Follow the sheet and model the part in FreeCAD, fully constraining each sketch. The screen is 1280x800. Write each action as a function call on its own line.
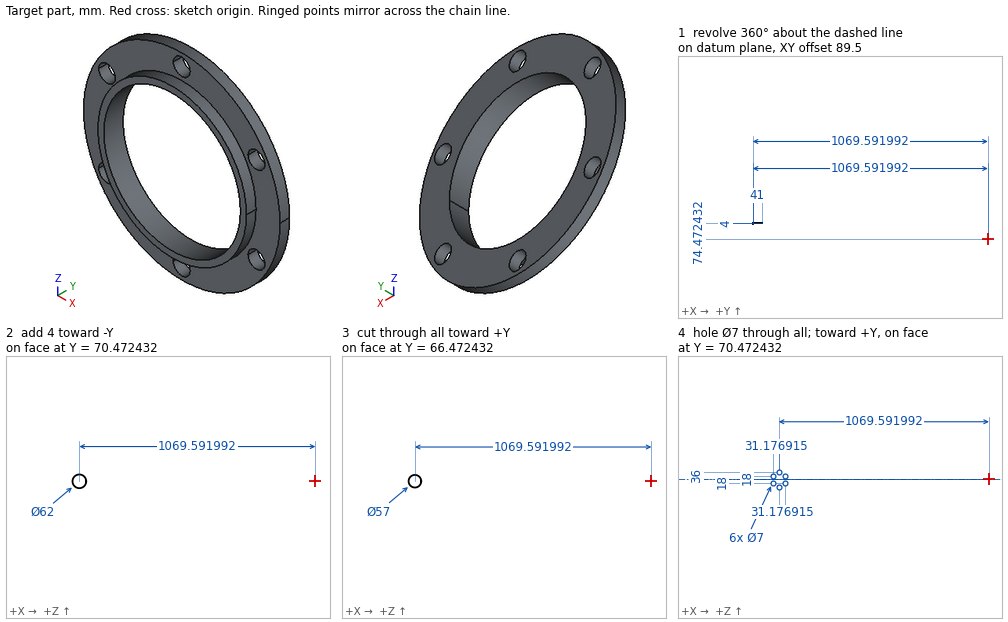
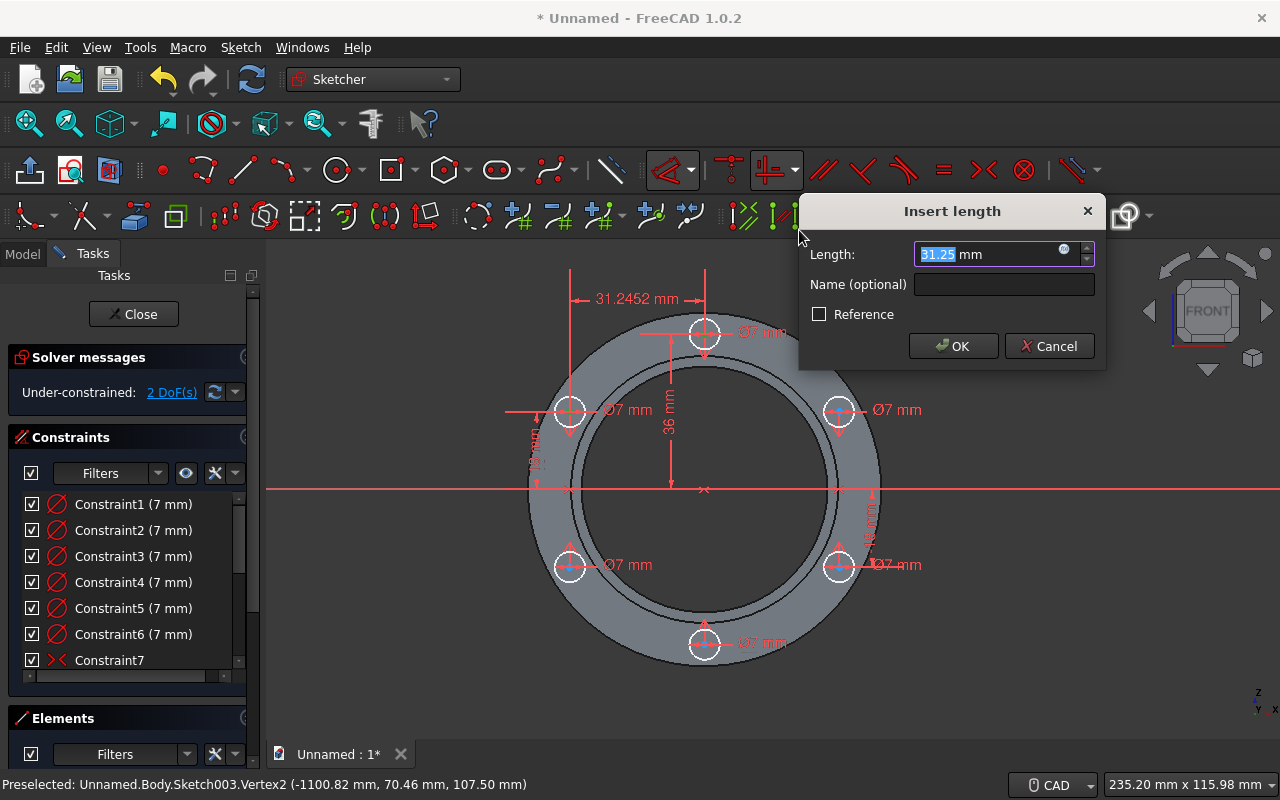
text(31.176915)
key(Return)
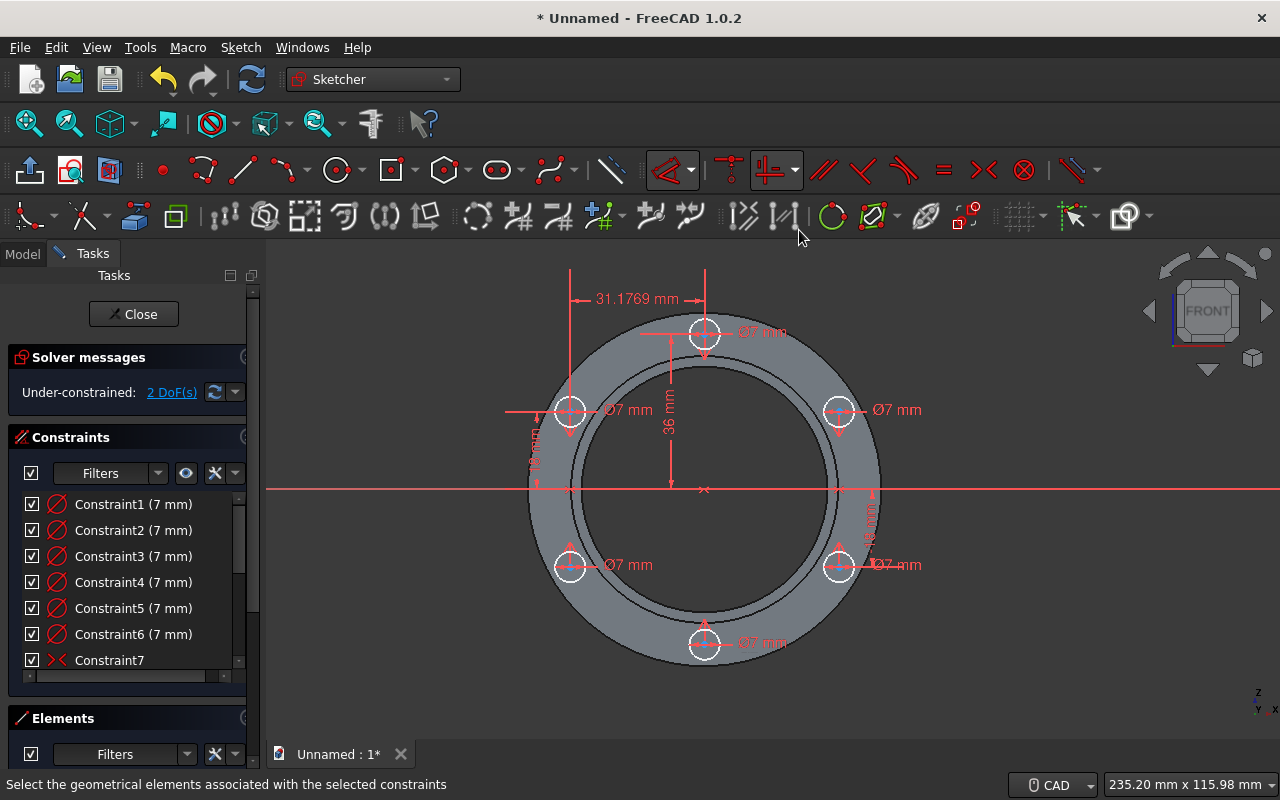
click(705, 645)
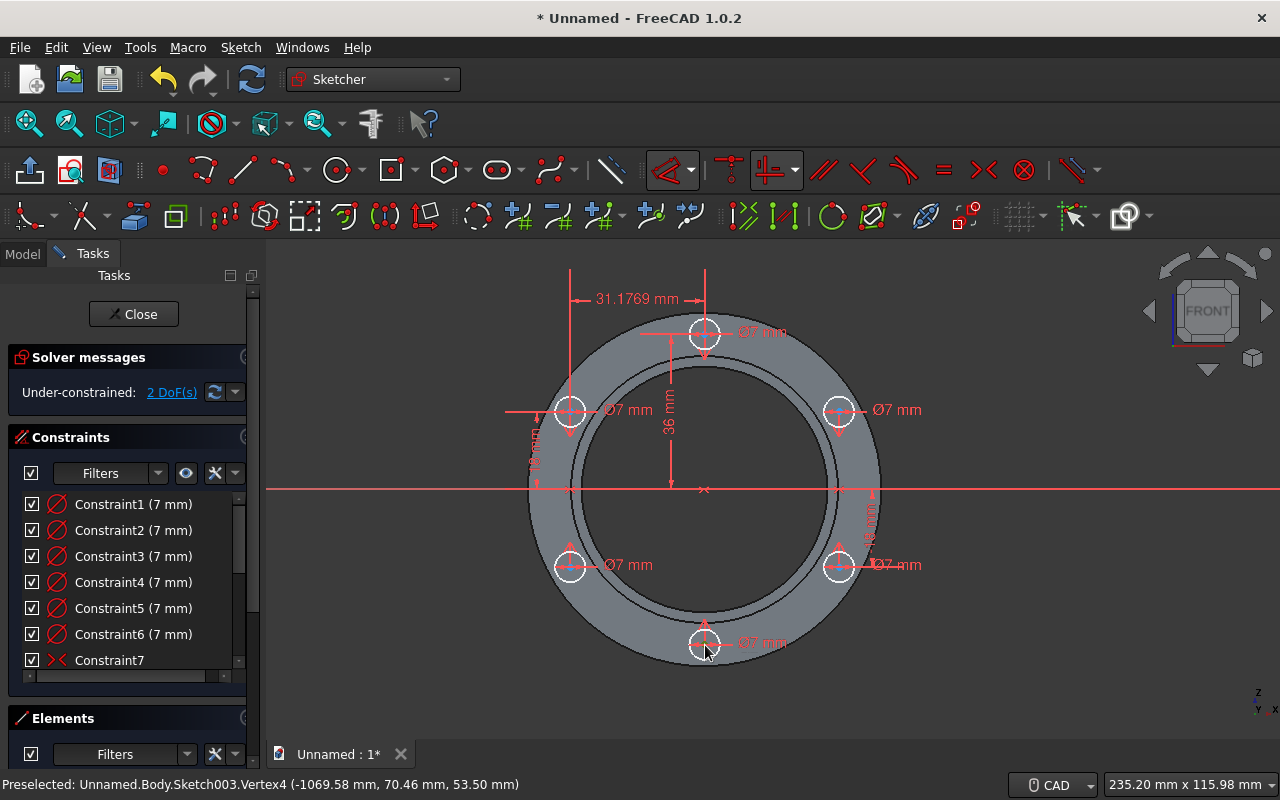
click(839, 567)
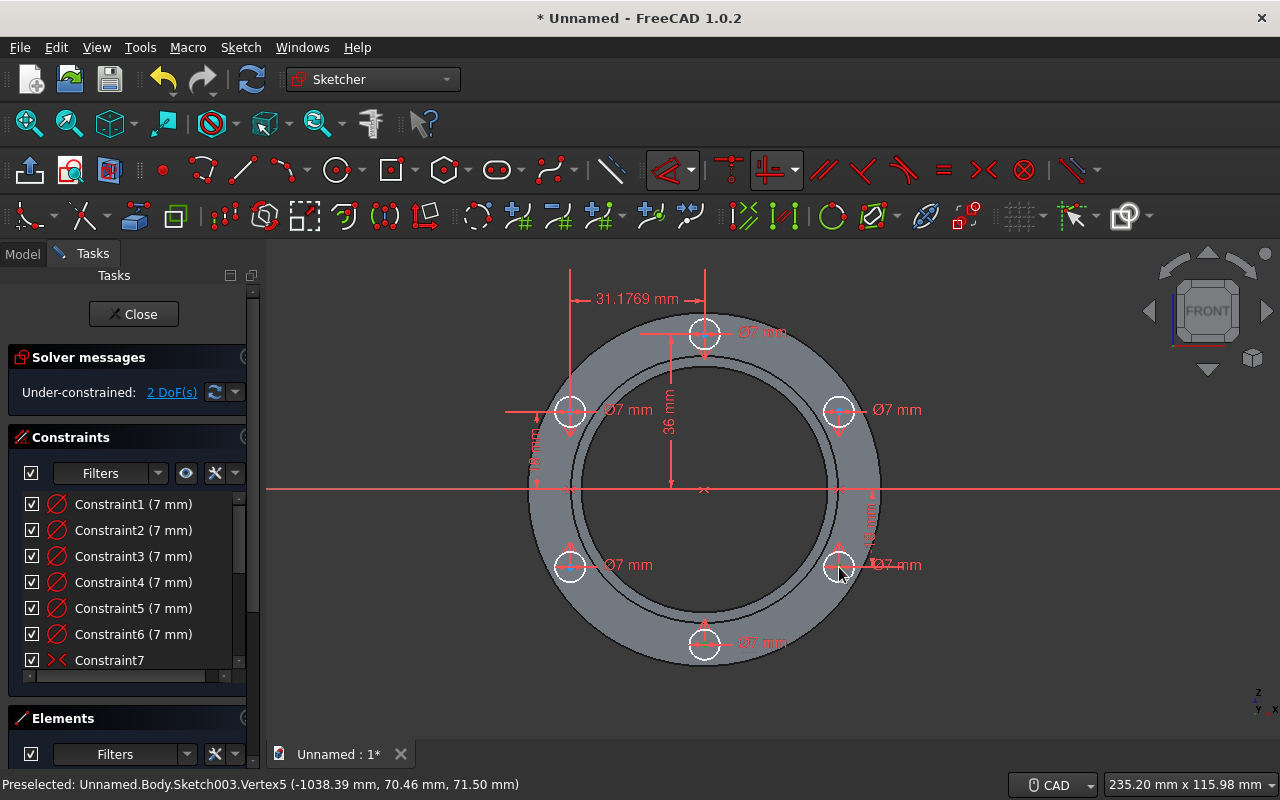
key(l)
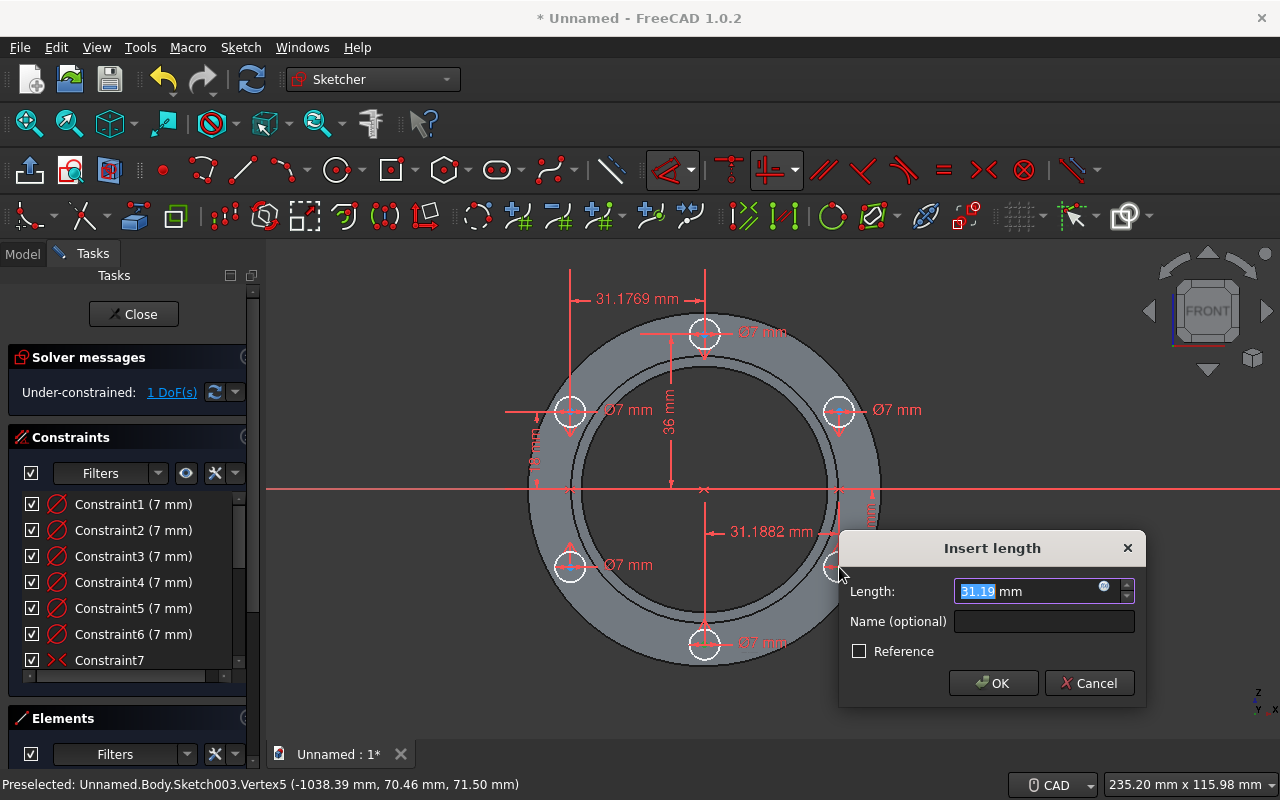
text(31.176915)
key(Return)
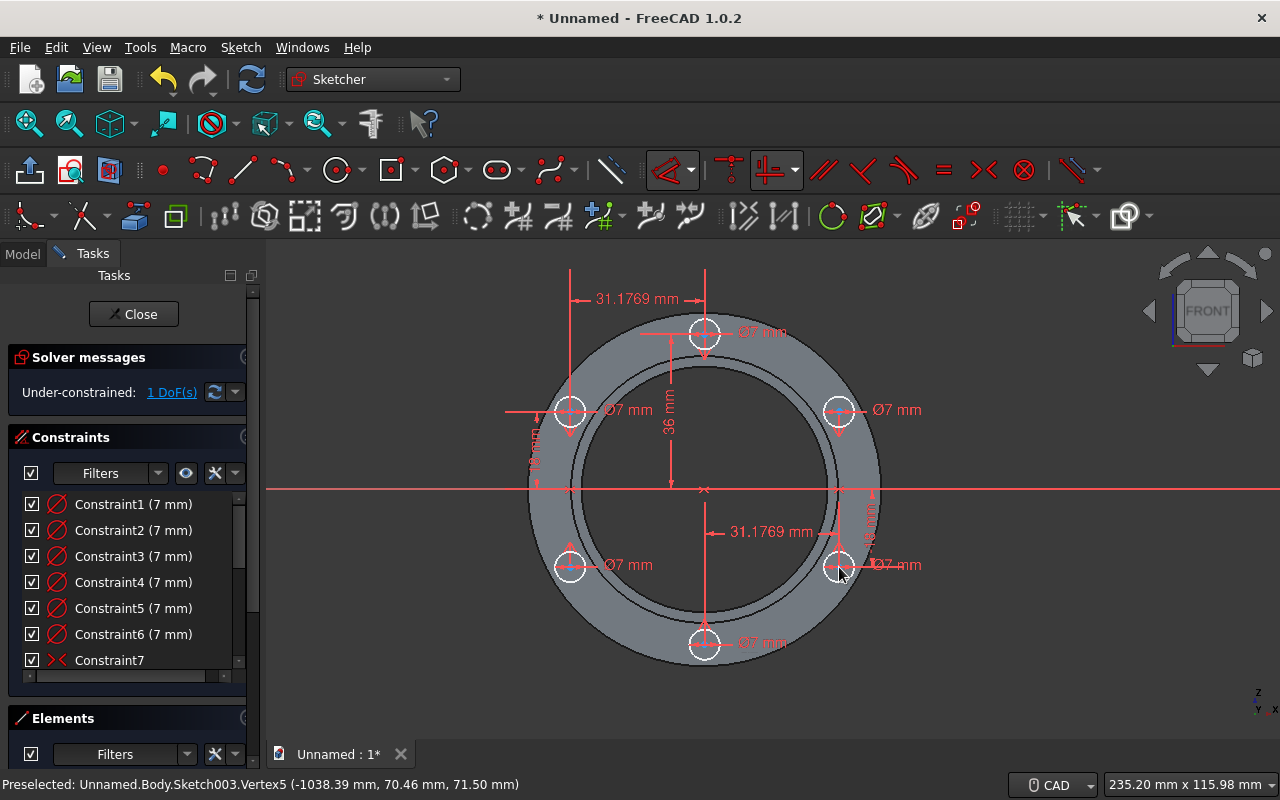
click(705, 334)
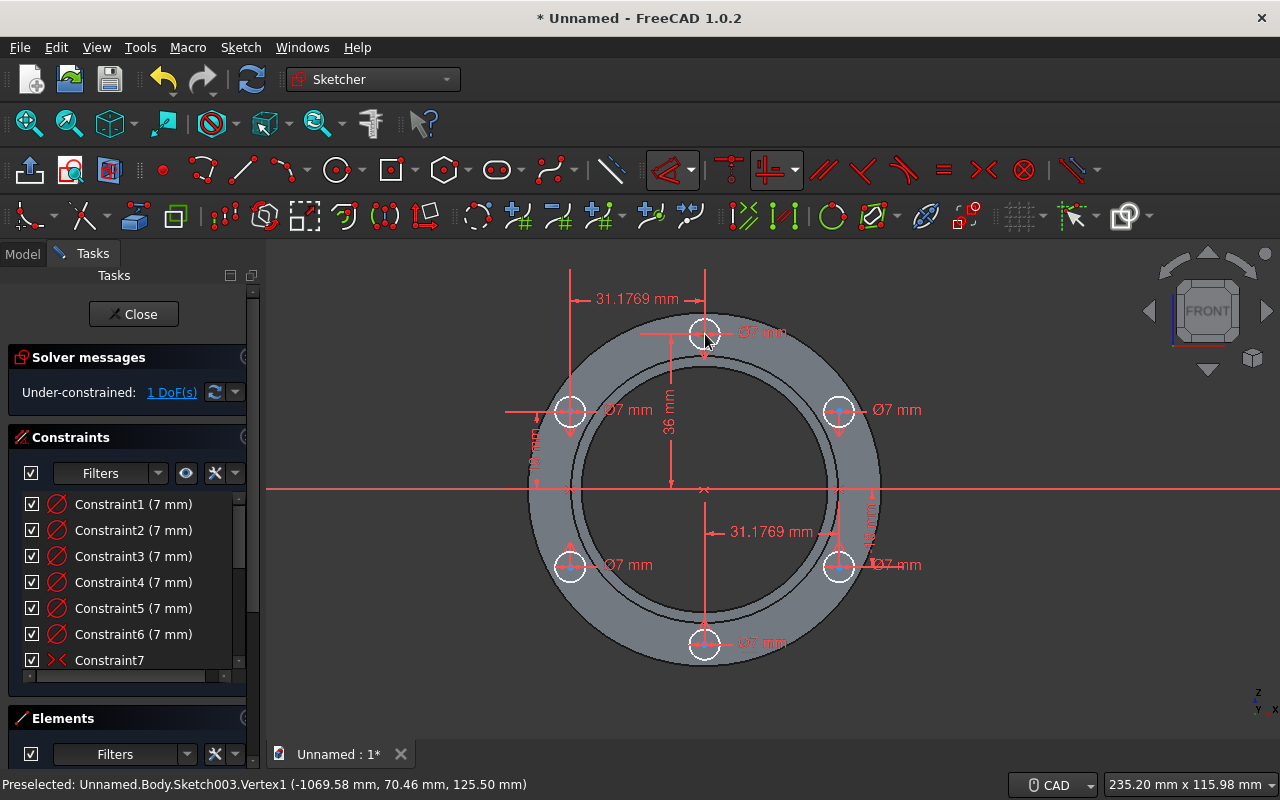
key(l)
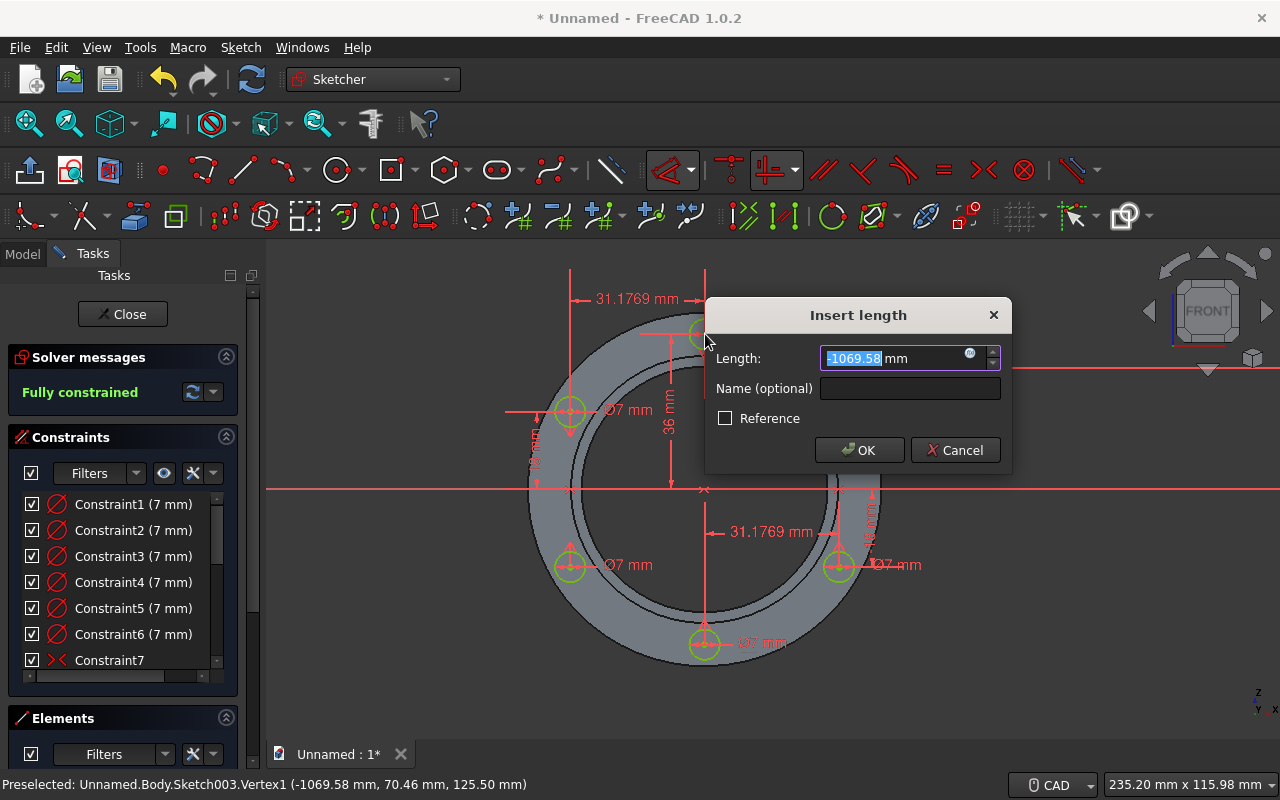
text(-1069.591992)
key(Return)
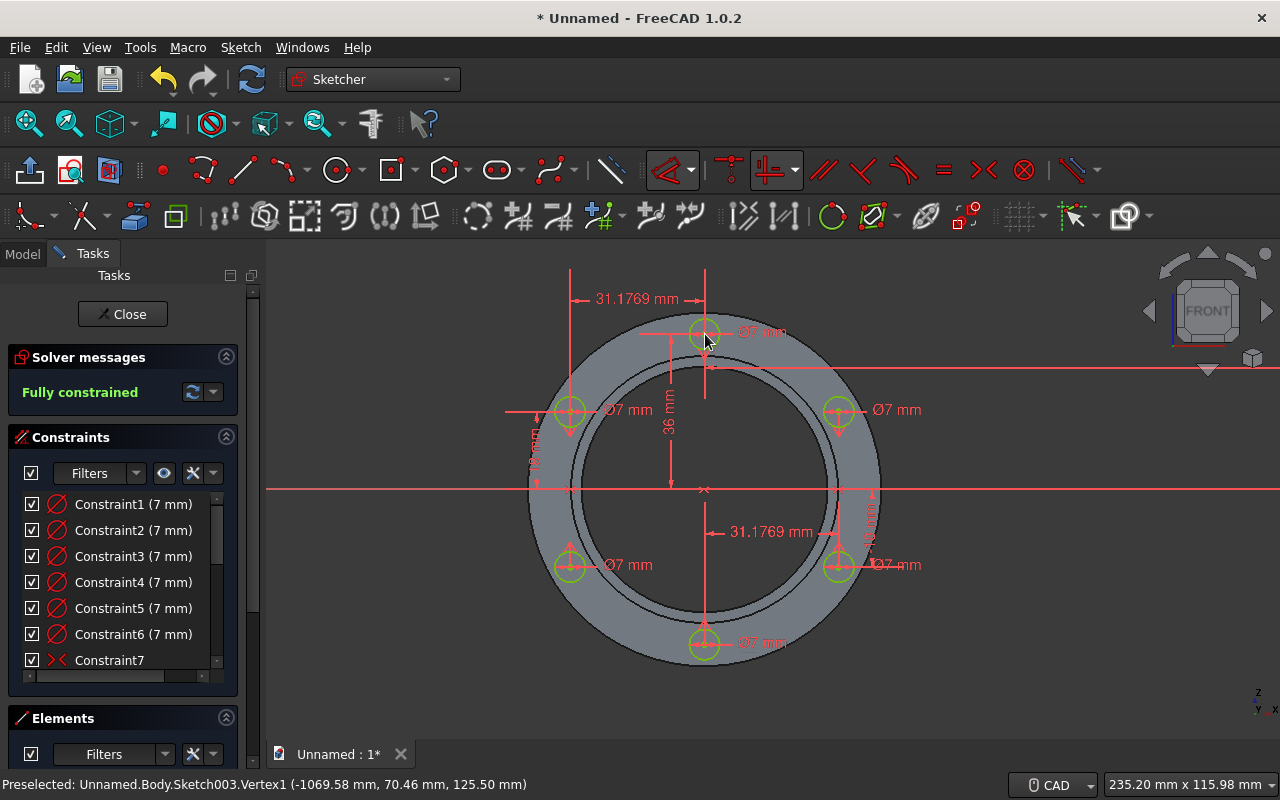
click(123, 314)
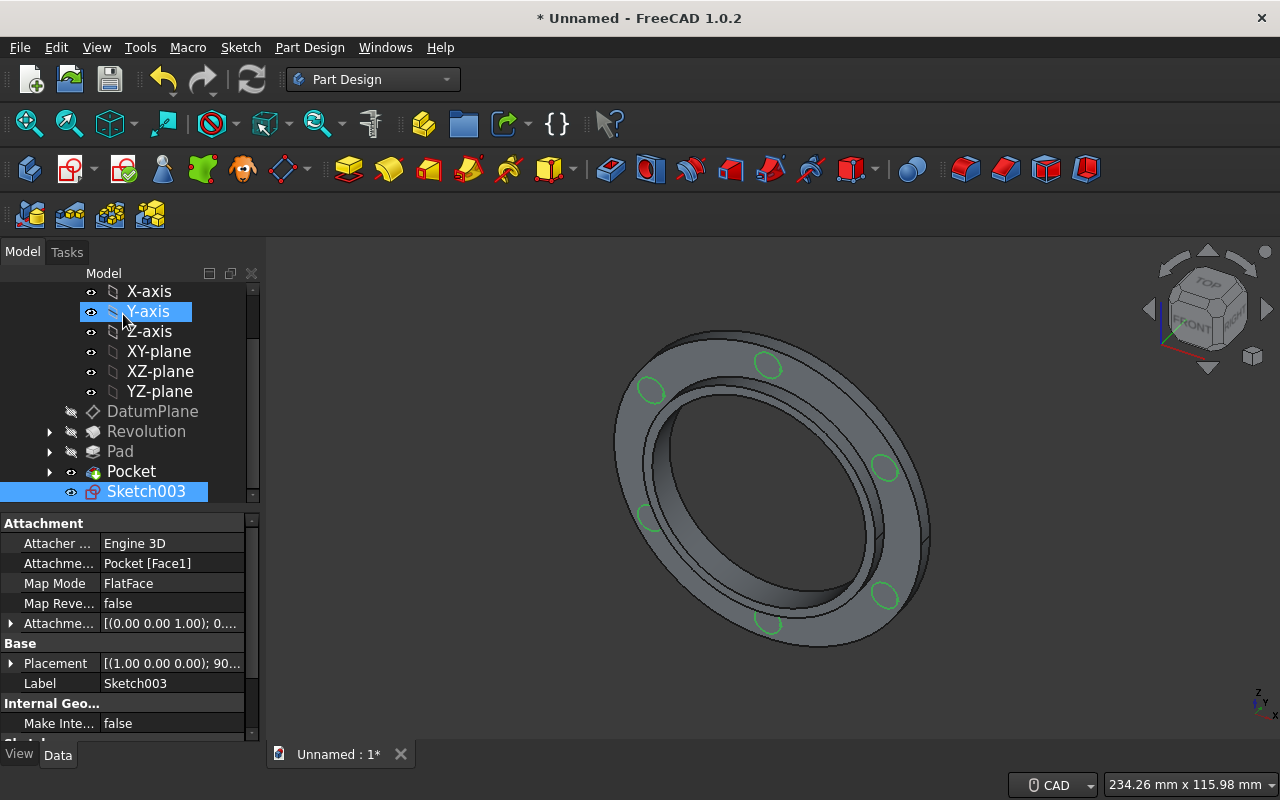
click(652, 170)